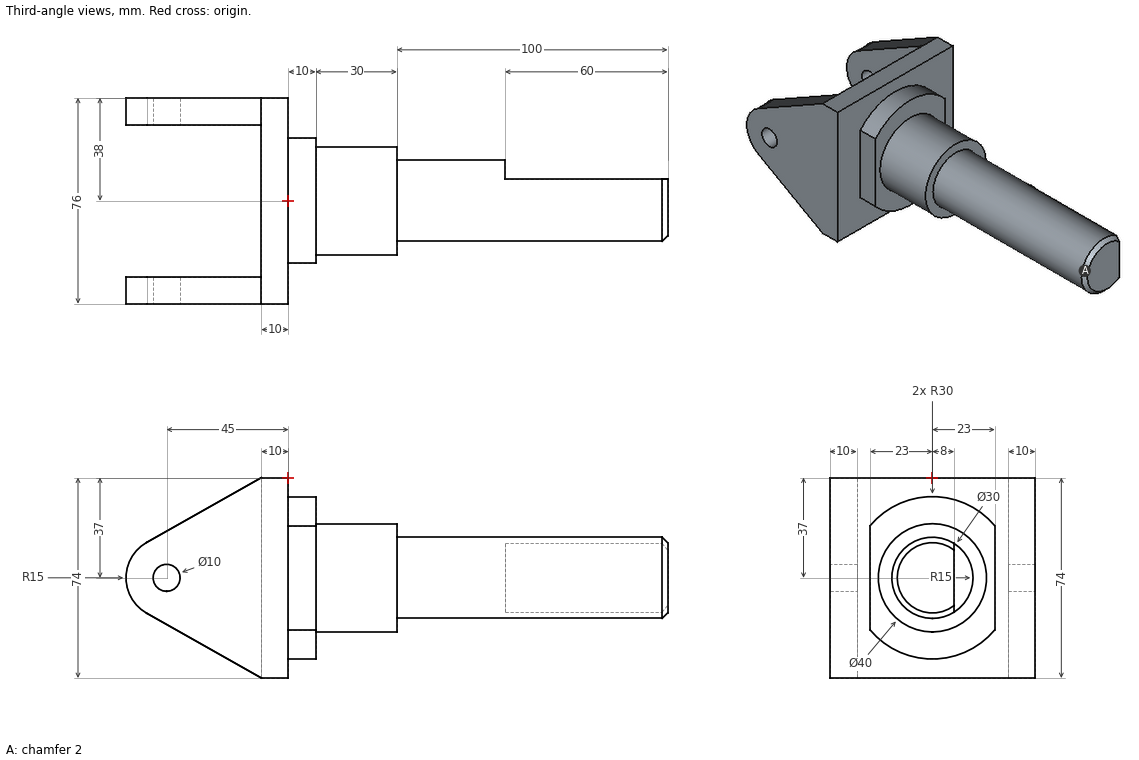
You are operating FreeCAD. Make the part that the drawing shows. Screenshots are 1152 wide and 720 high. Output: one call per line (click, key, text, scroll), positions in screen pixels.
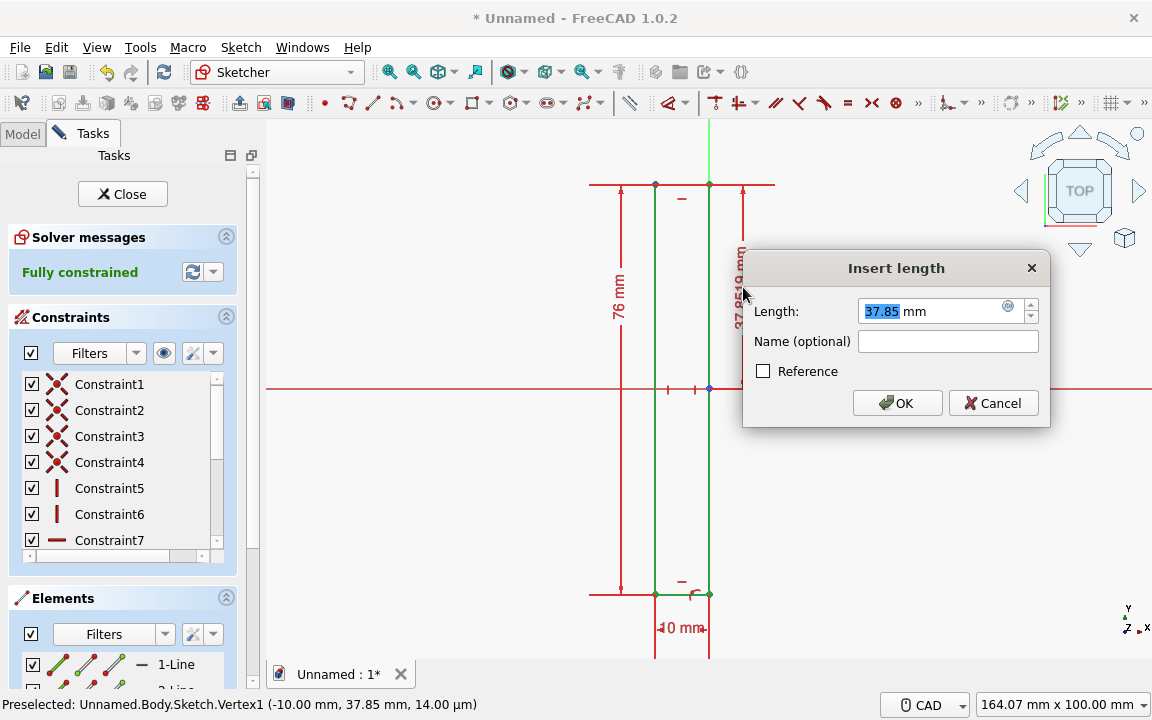
text(38)
key(Return)
key(Escape)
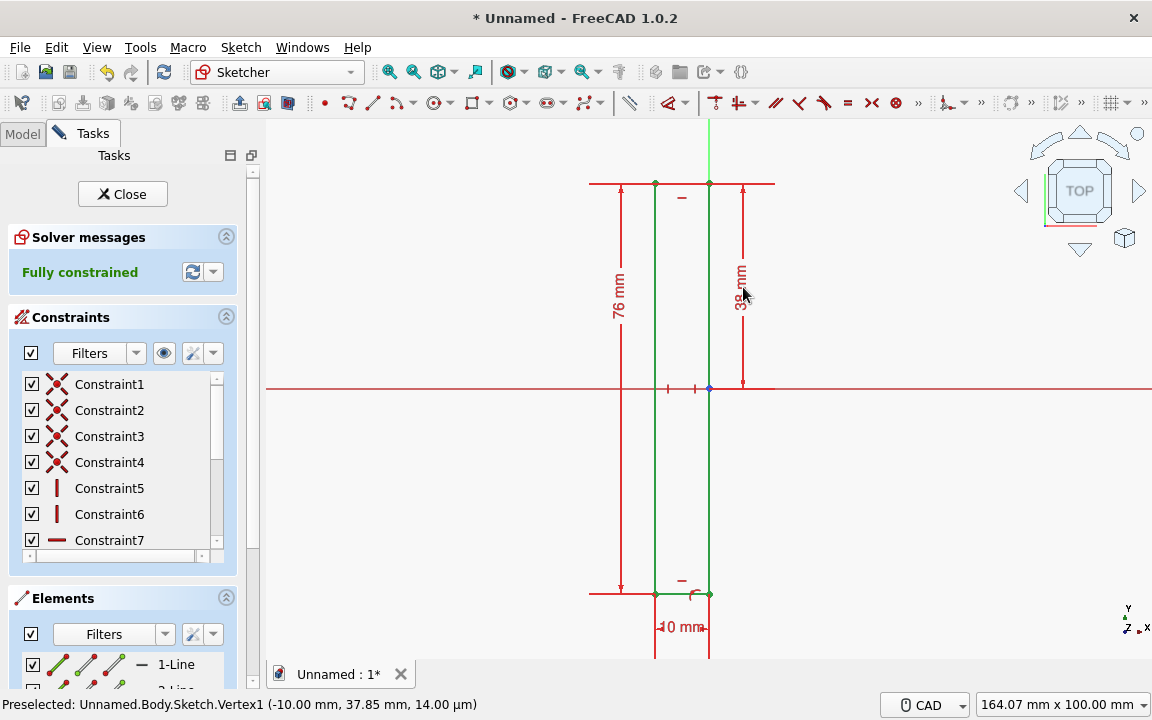
click(123, 194)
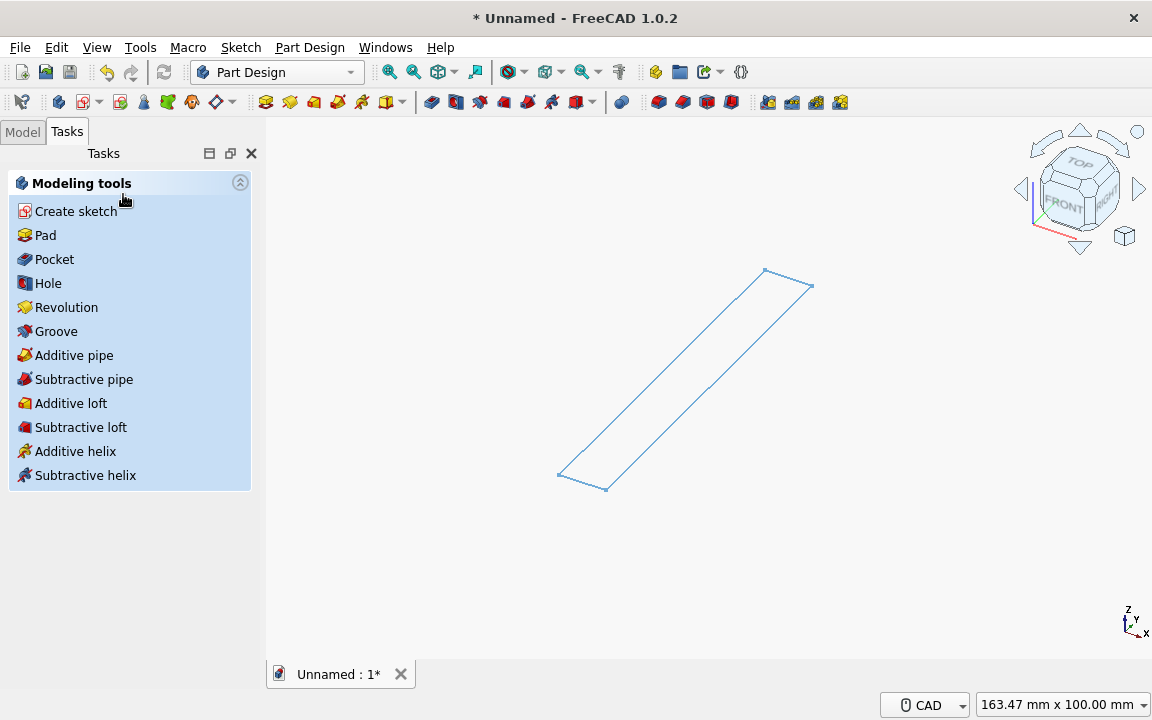
click(266, 102)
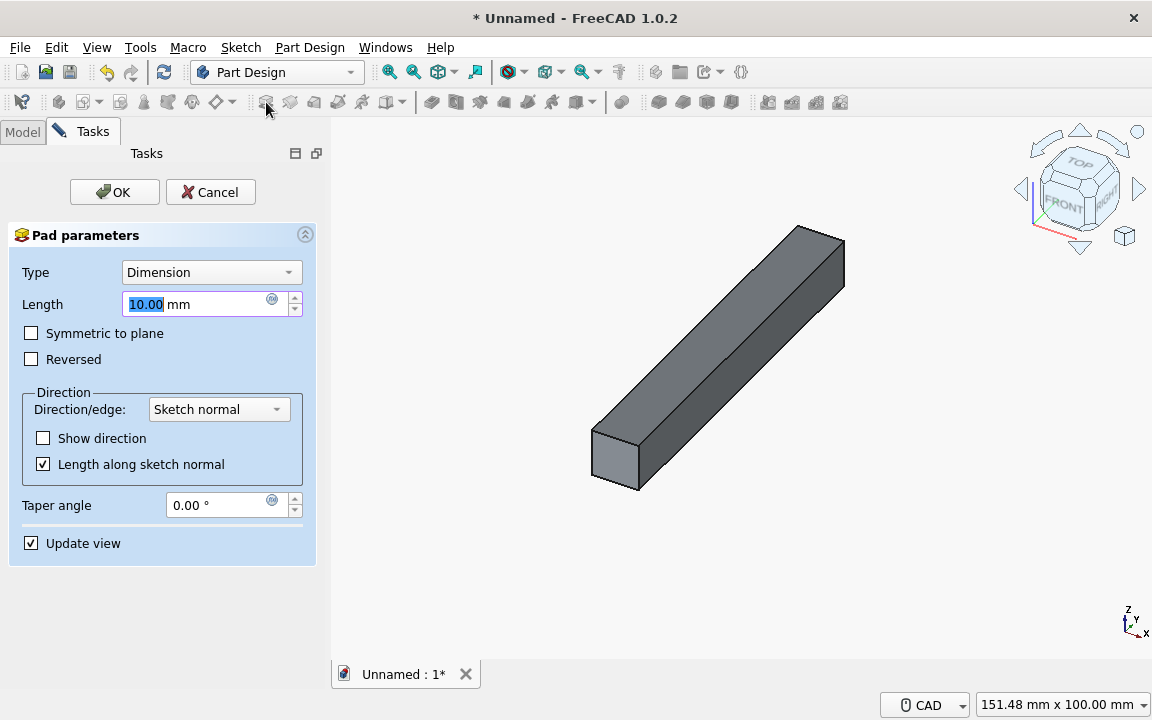
text(74)
key(Tab)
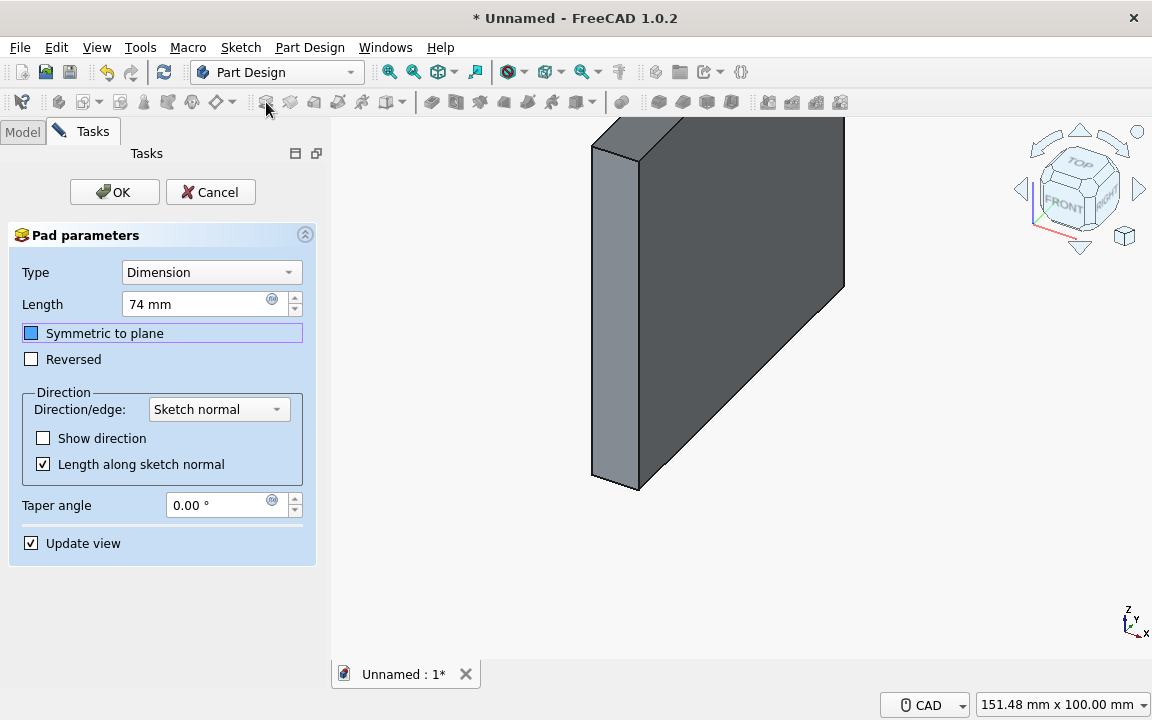
click(30, 359)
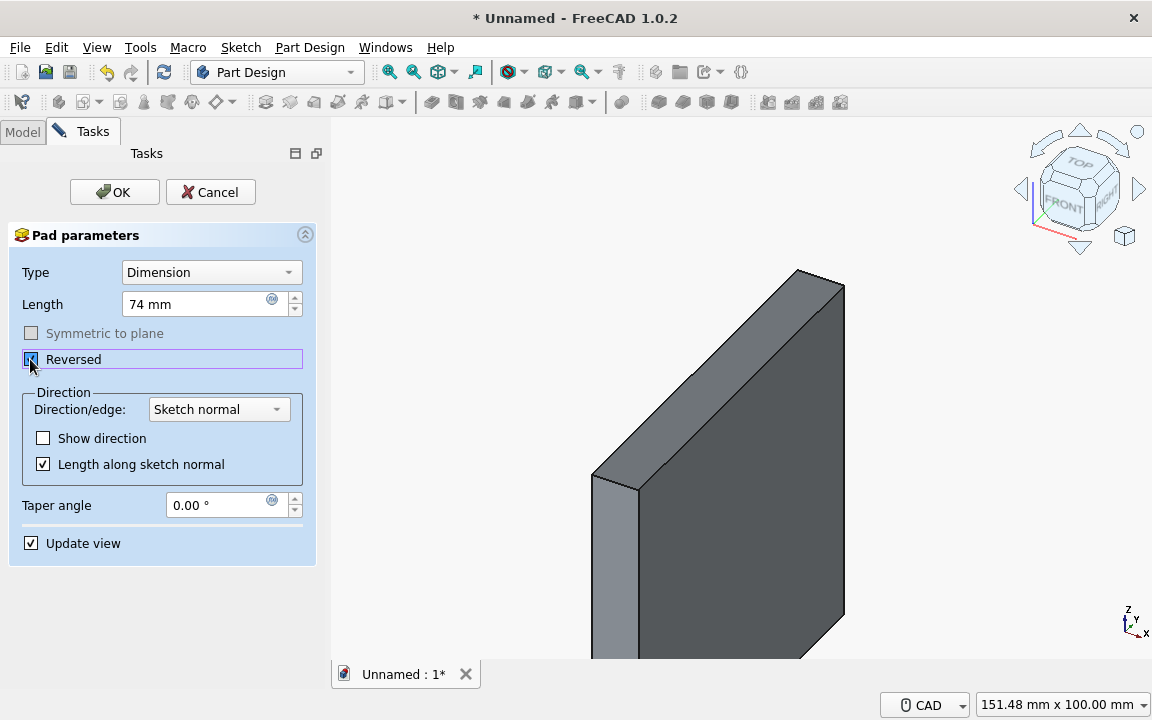
click(115, 192)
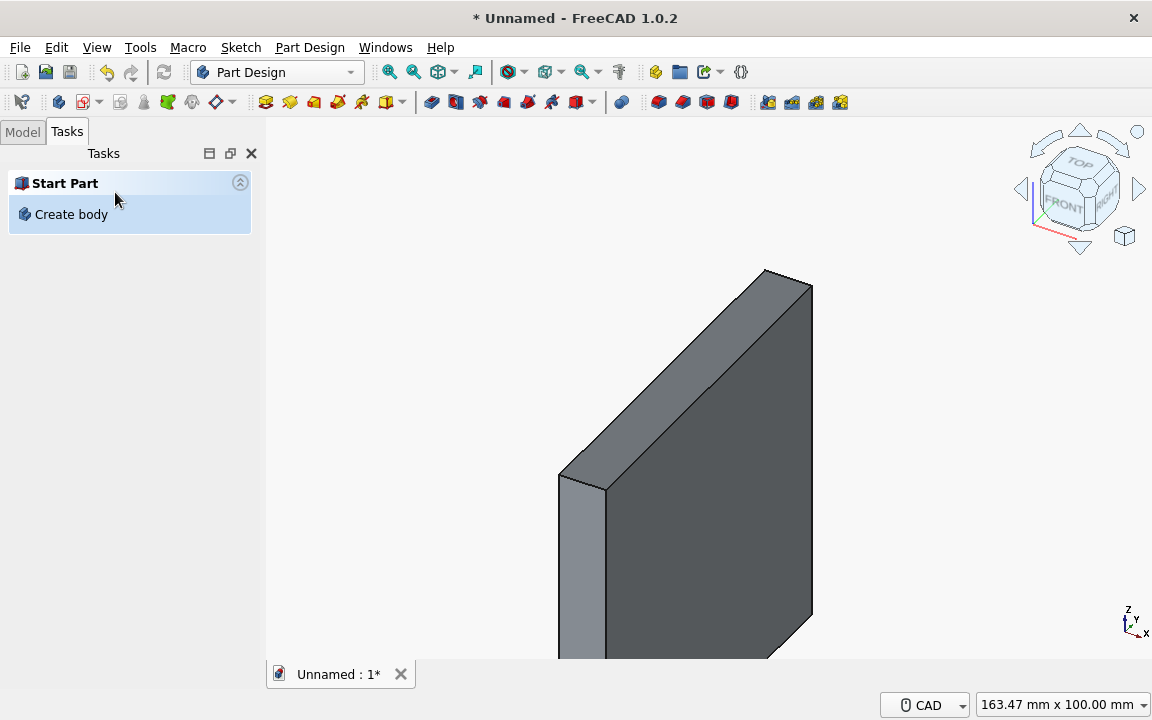
click(390, 72)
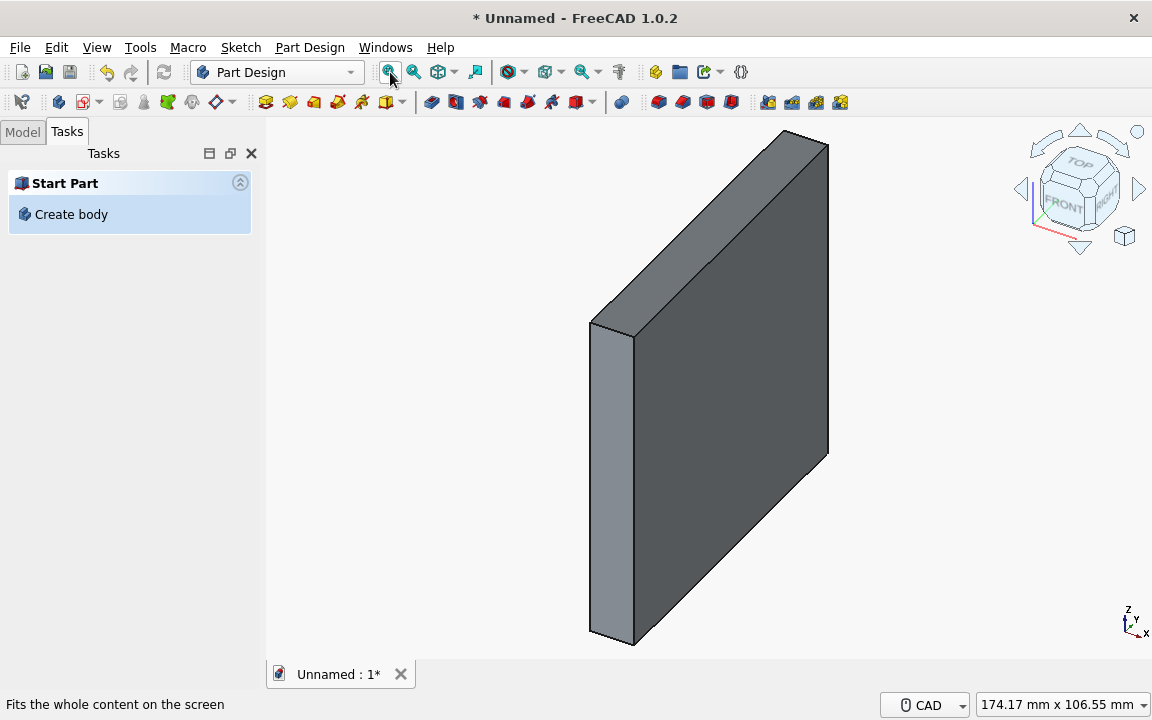
key(4)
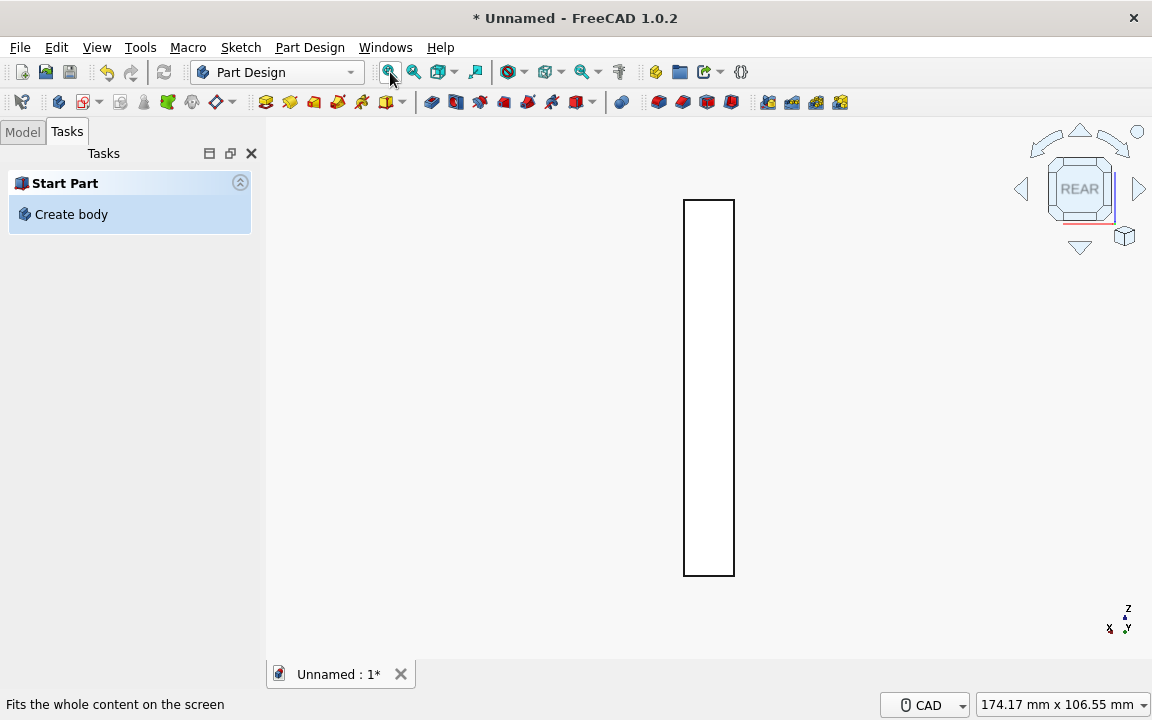
click(709, 226)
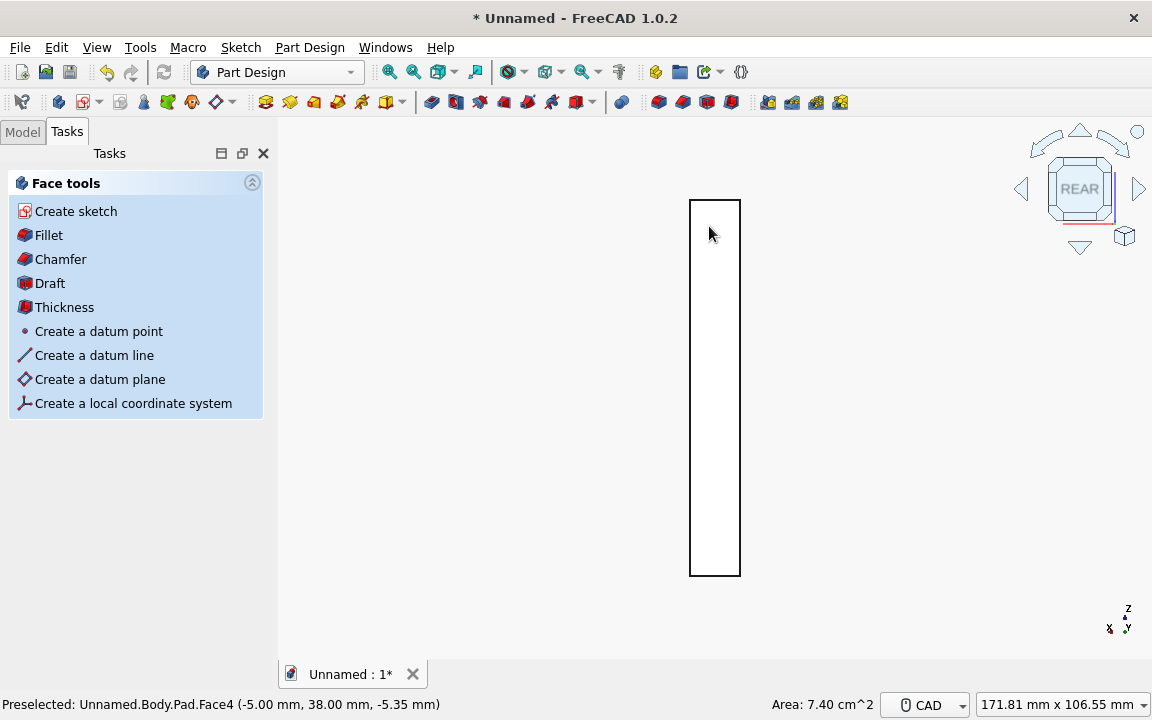
click(84, 102)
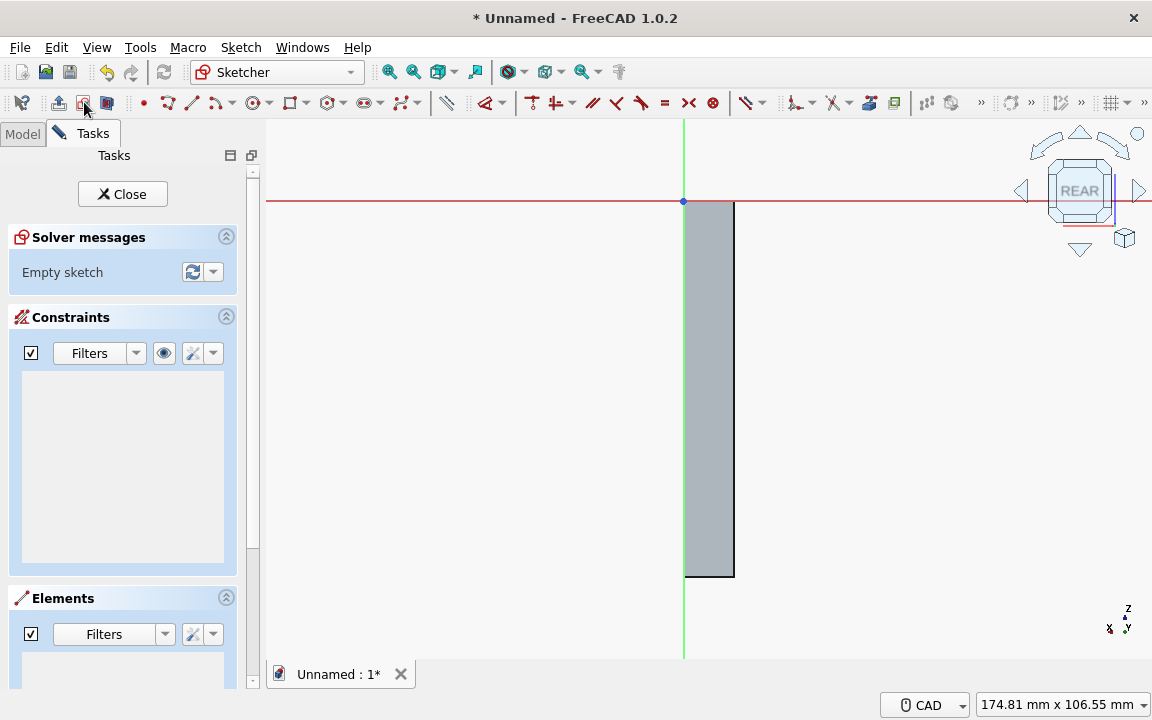
scroll(294, 389, down, 1)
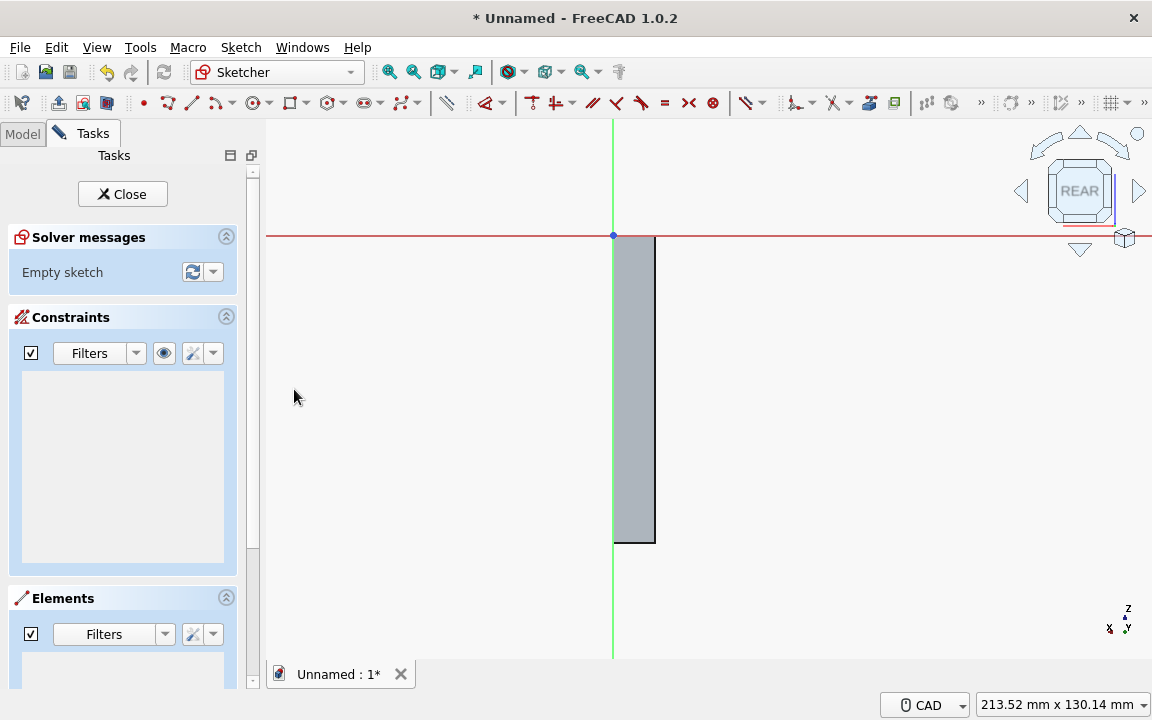
click(168, 104)